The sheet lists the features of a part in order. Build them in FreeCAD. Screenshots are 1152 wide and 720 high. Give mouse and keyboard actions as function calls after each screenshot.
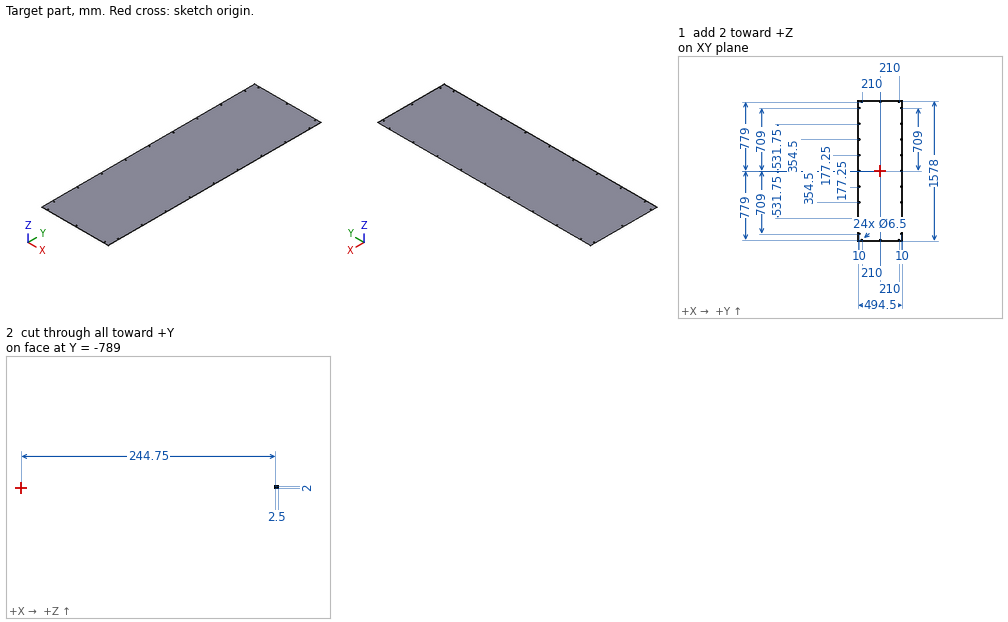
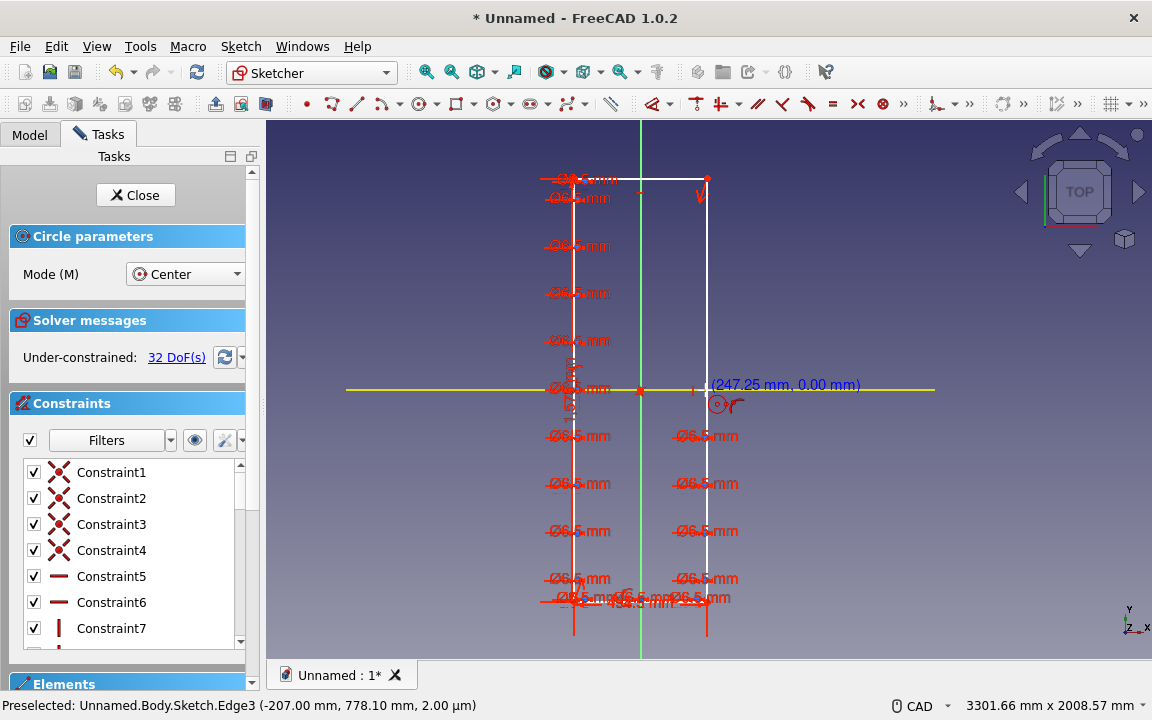
scroll(704, 390, up, 9)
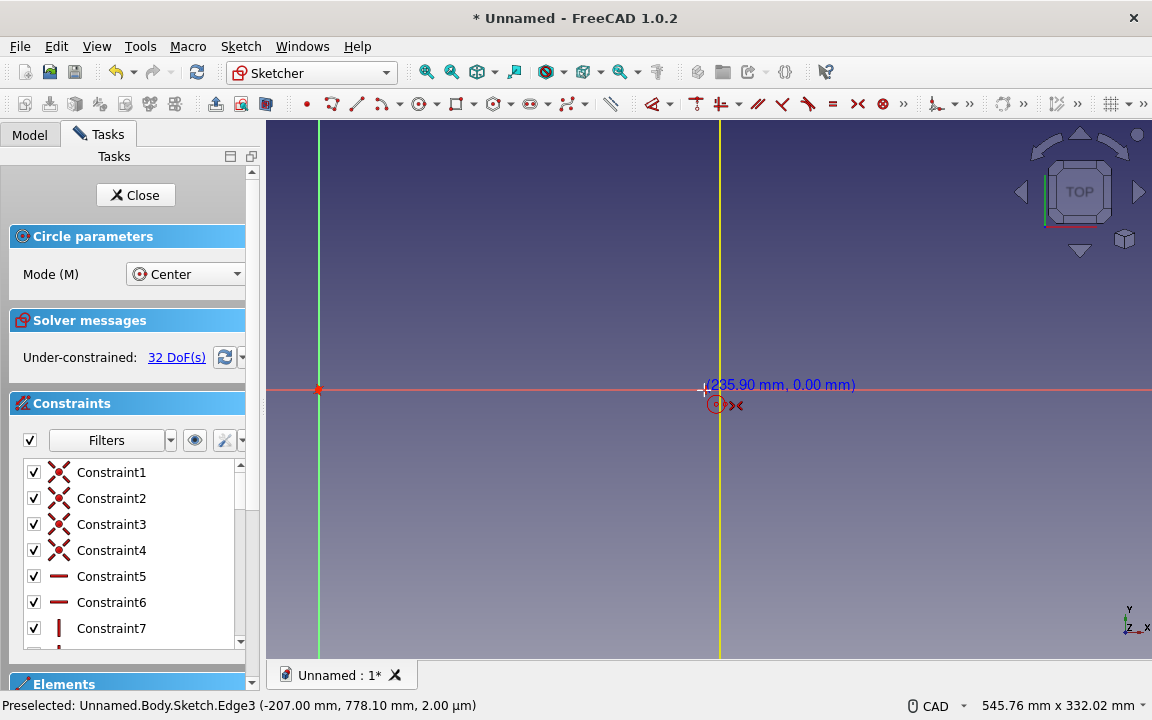
click(704, 390)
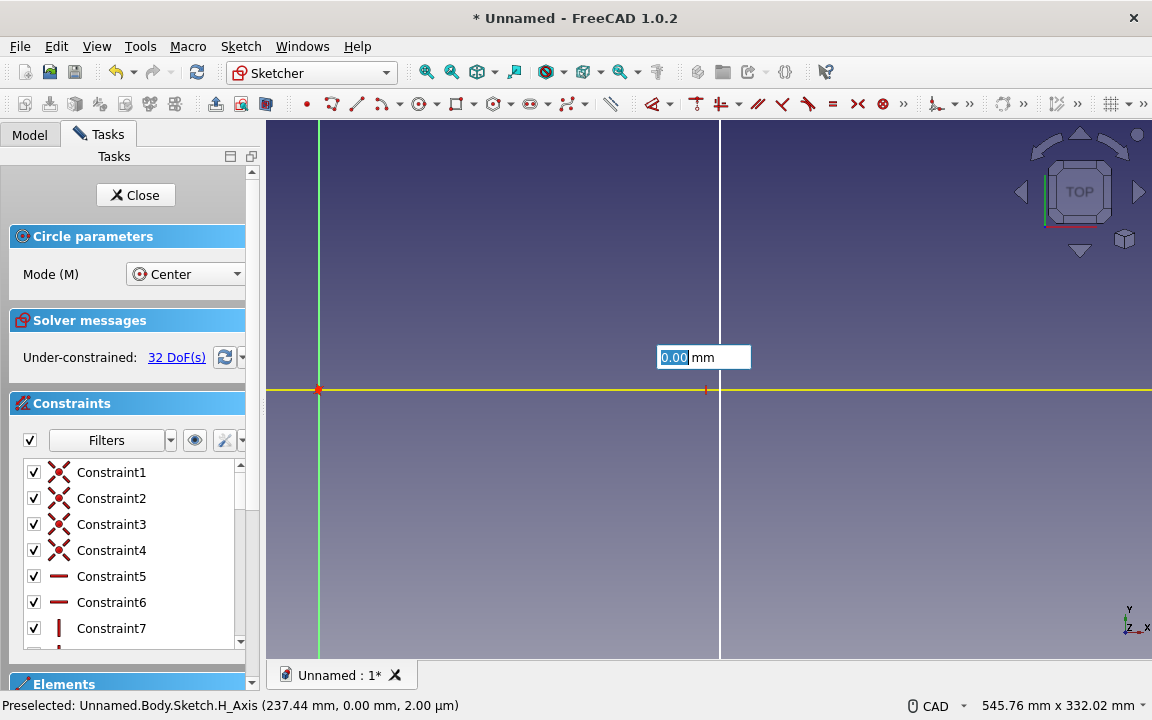
scroll(702, 395, up, 6)
move(700, 393)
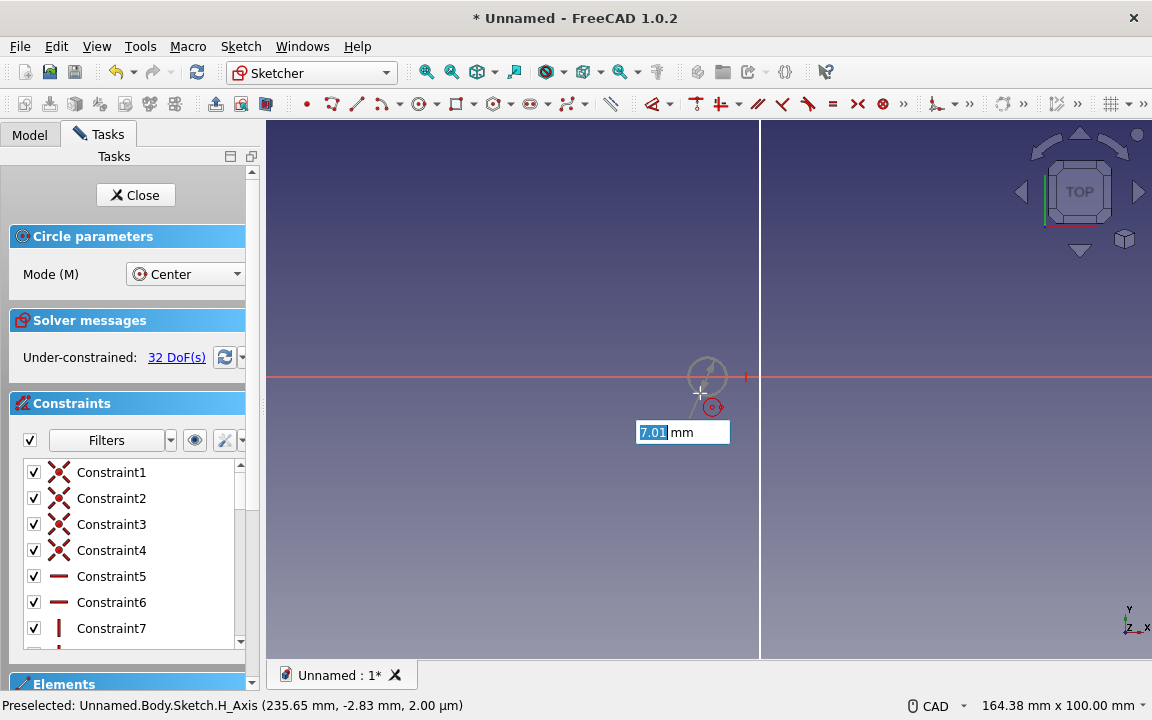
text(6.5)
key(Return)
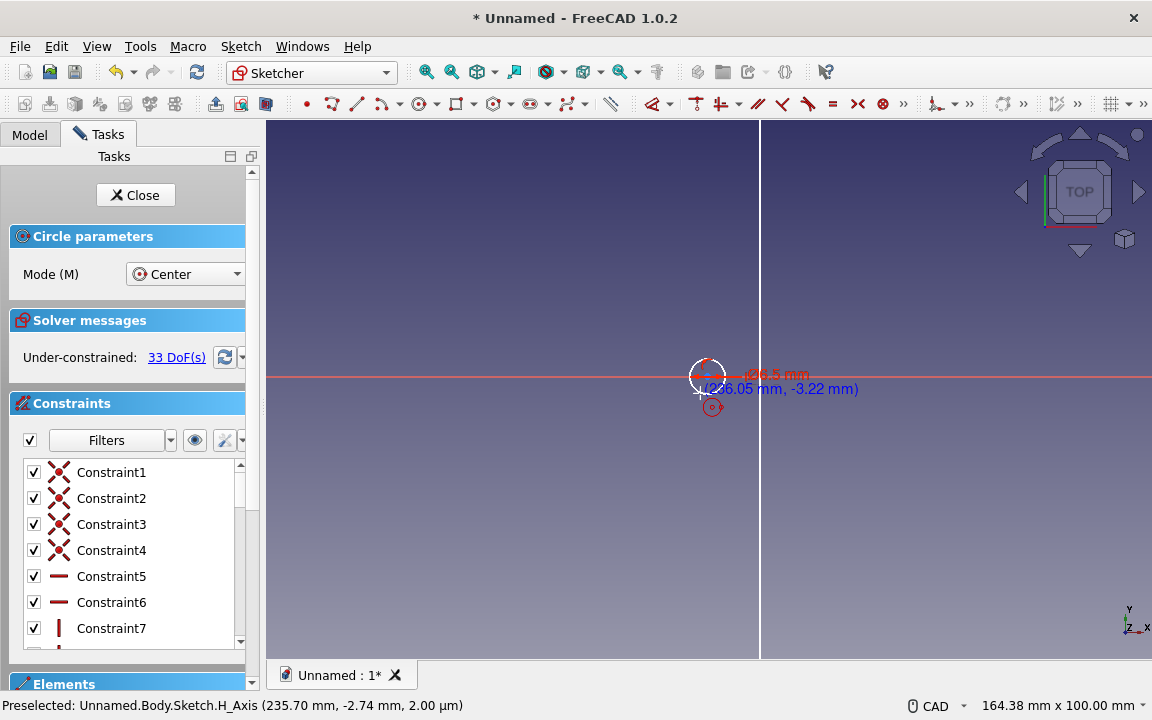
scroll(704, 390, down, 15)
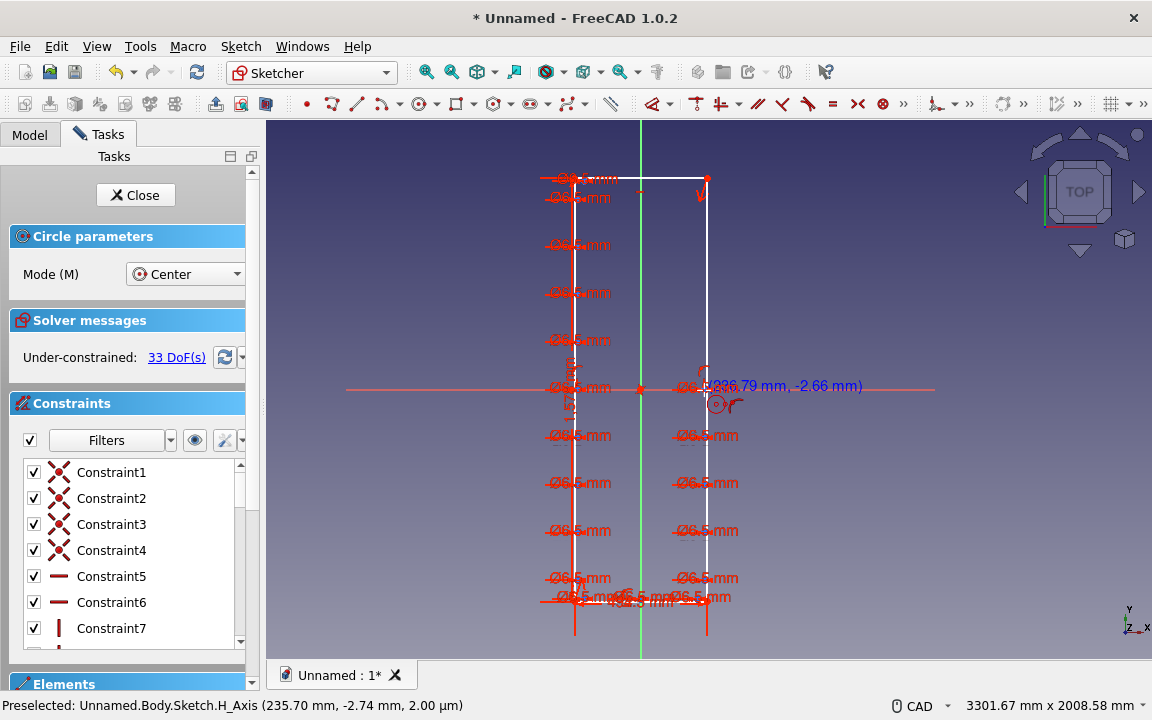
scroll(705, 342, up, 17)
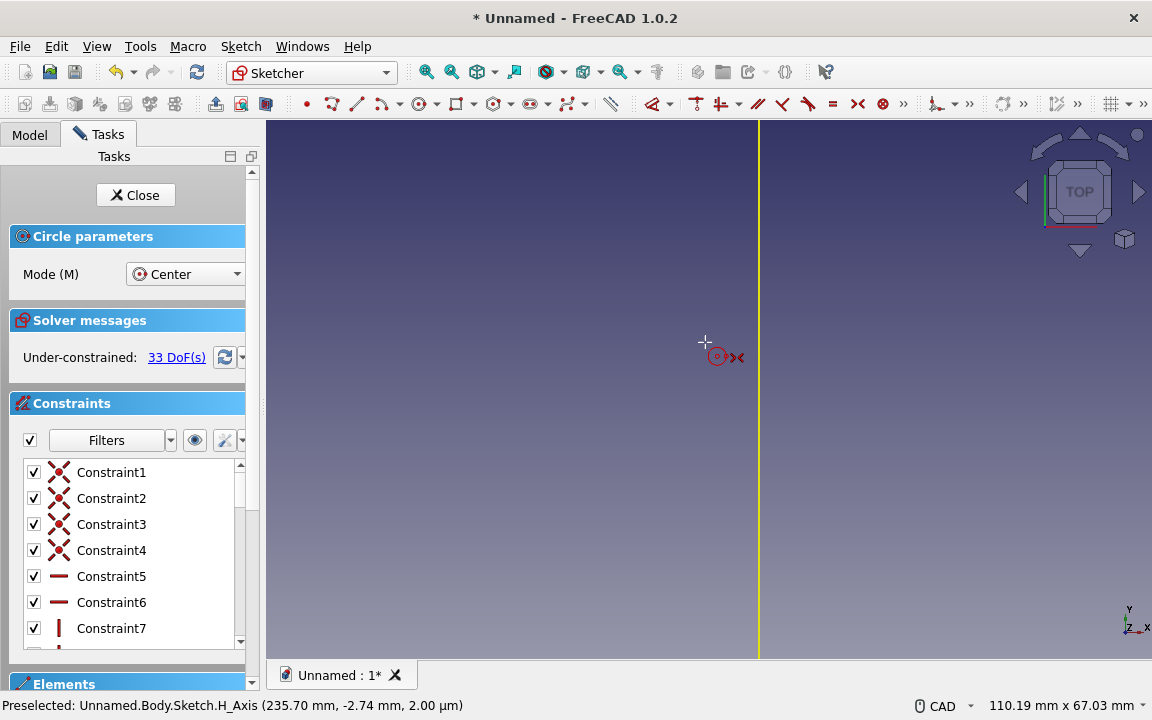
scroll(705, 342, down, 17)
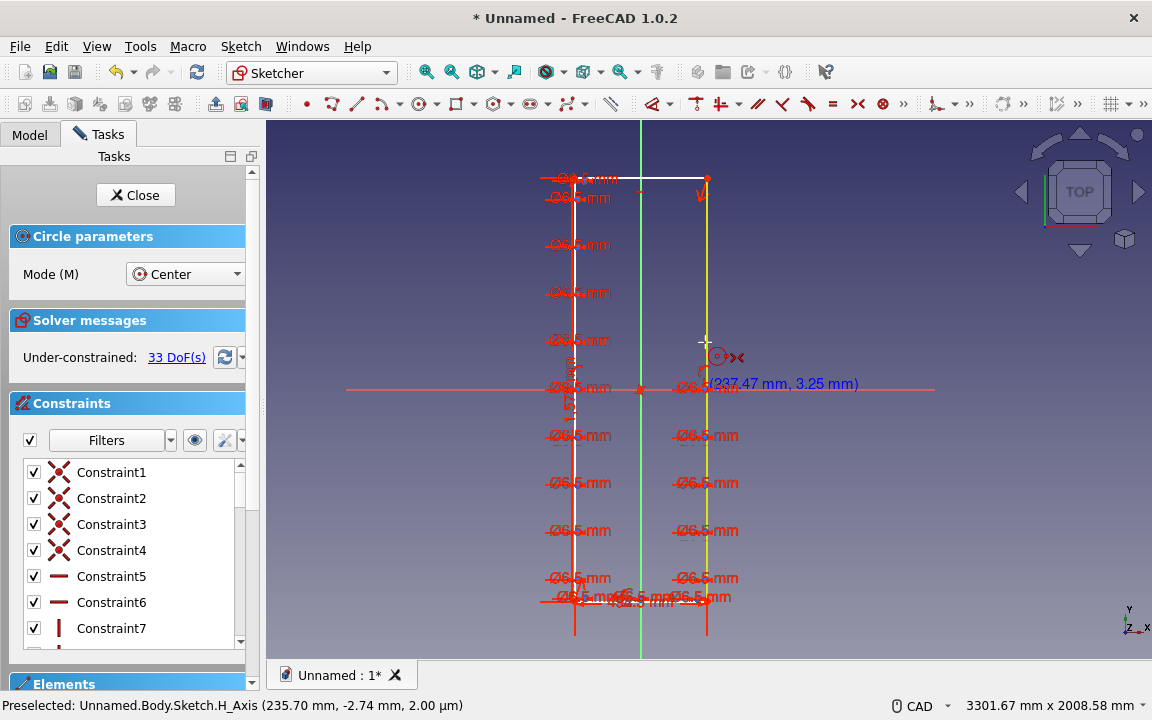
scroll(705, 342, up, 9)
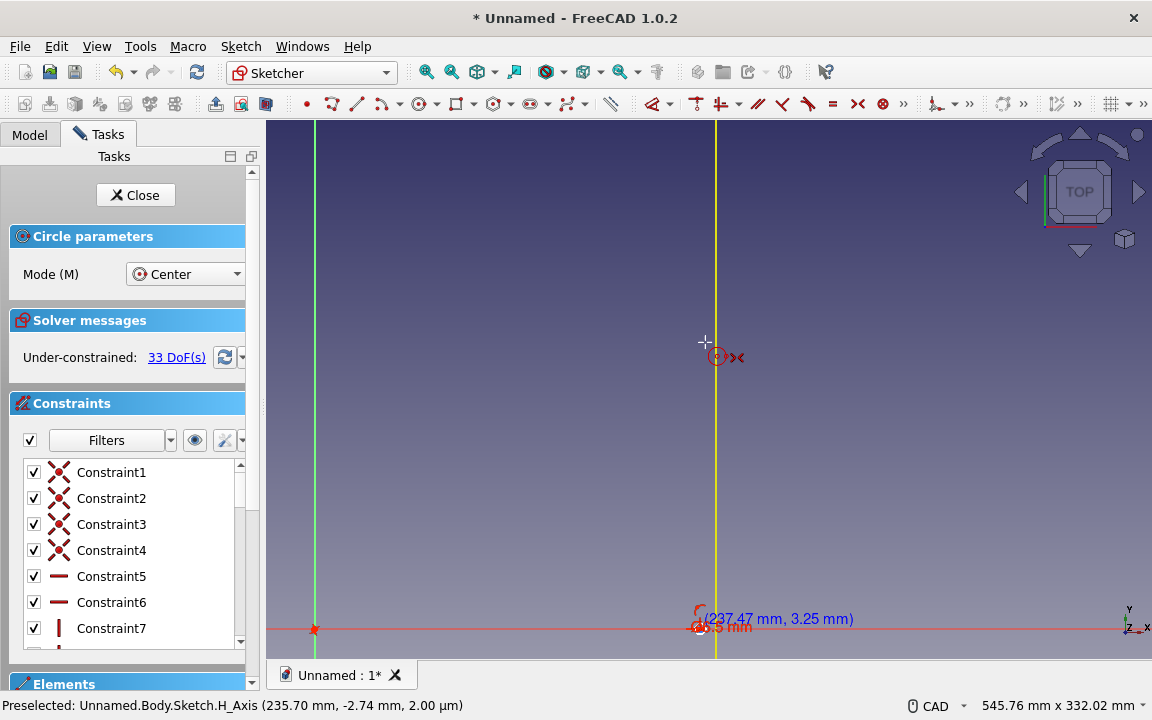
click(700, 341)
move(696, 338)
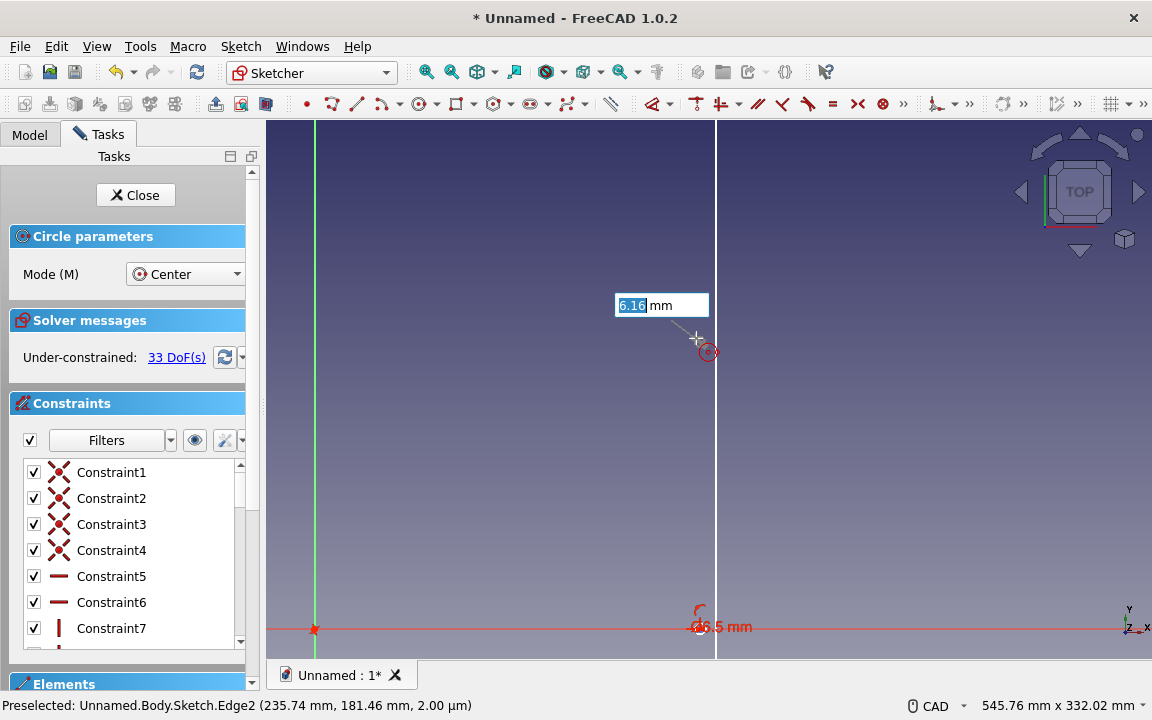
text(6.5)
key(Return)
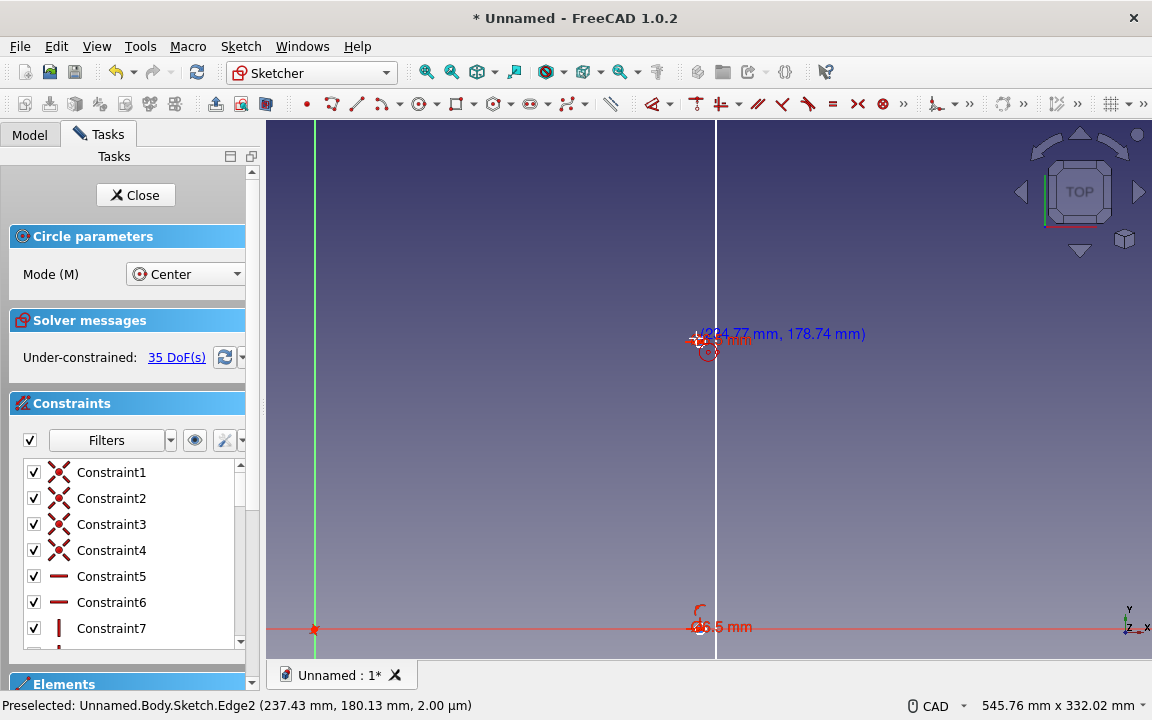
scroll(691, 352, down, 10)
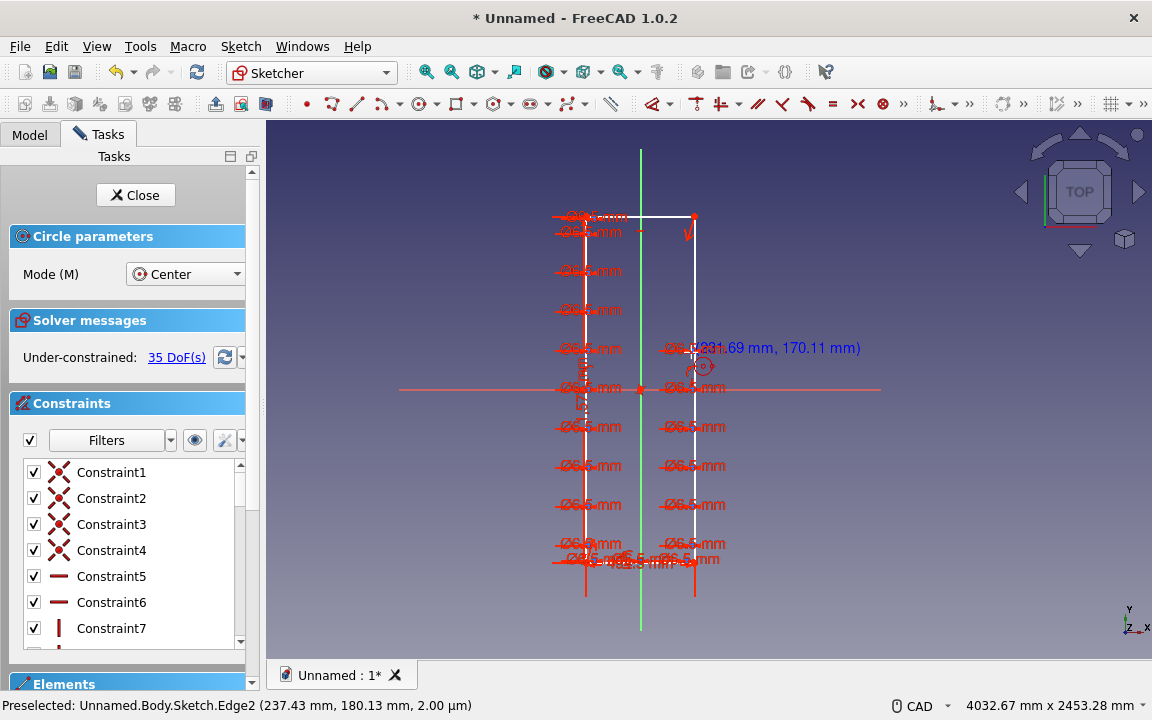
scroll(693, 312, up, 18)